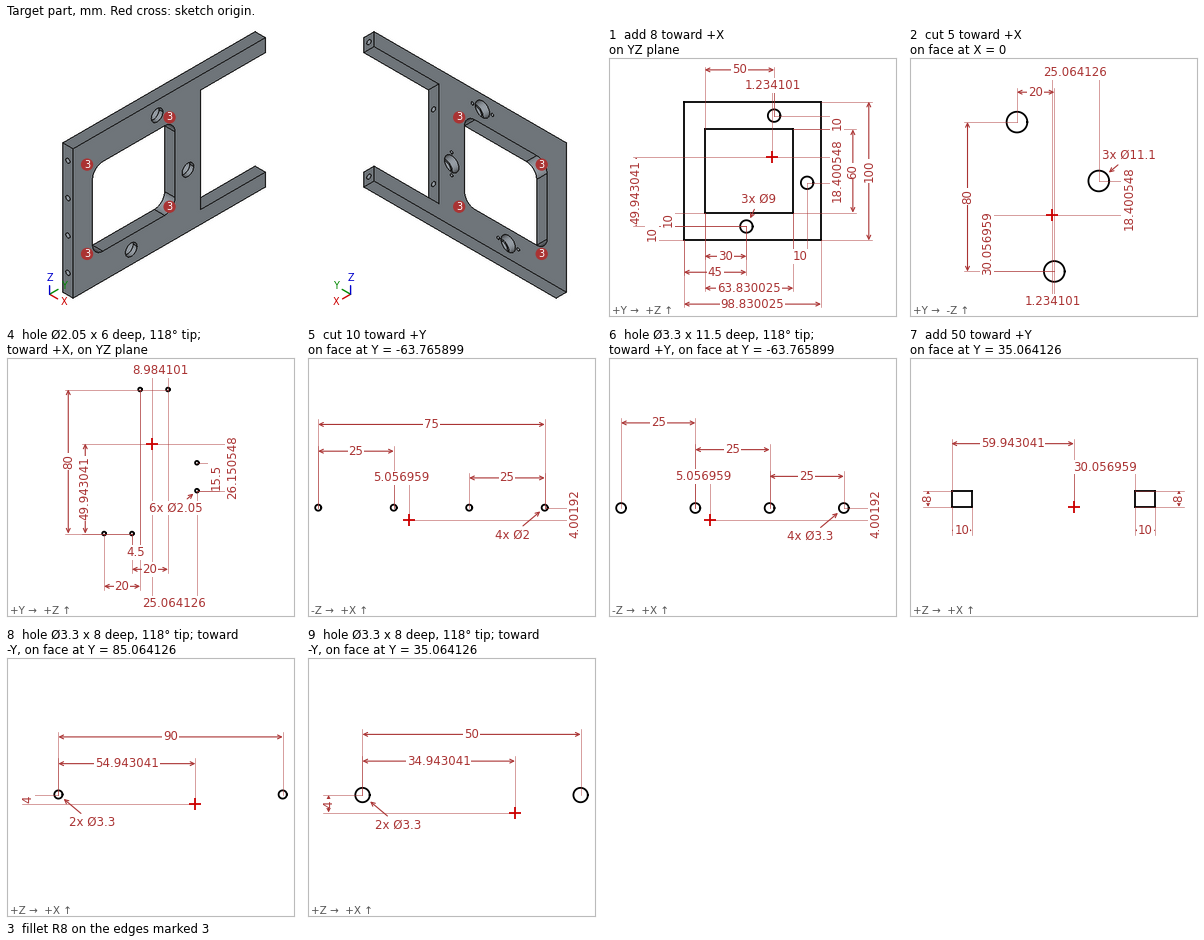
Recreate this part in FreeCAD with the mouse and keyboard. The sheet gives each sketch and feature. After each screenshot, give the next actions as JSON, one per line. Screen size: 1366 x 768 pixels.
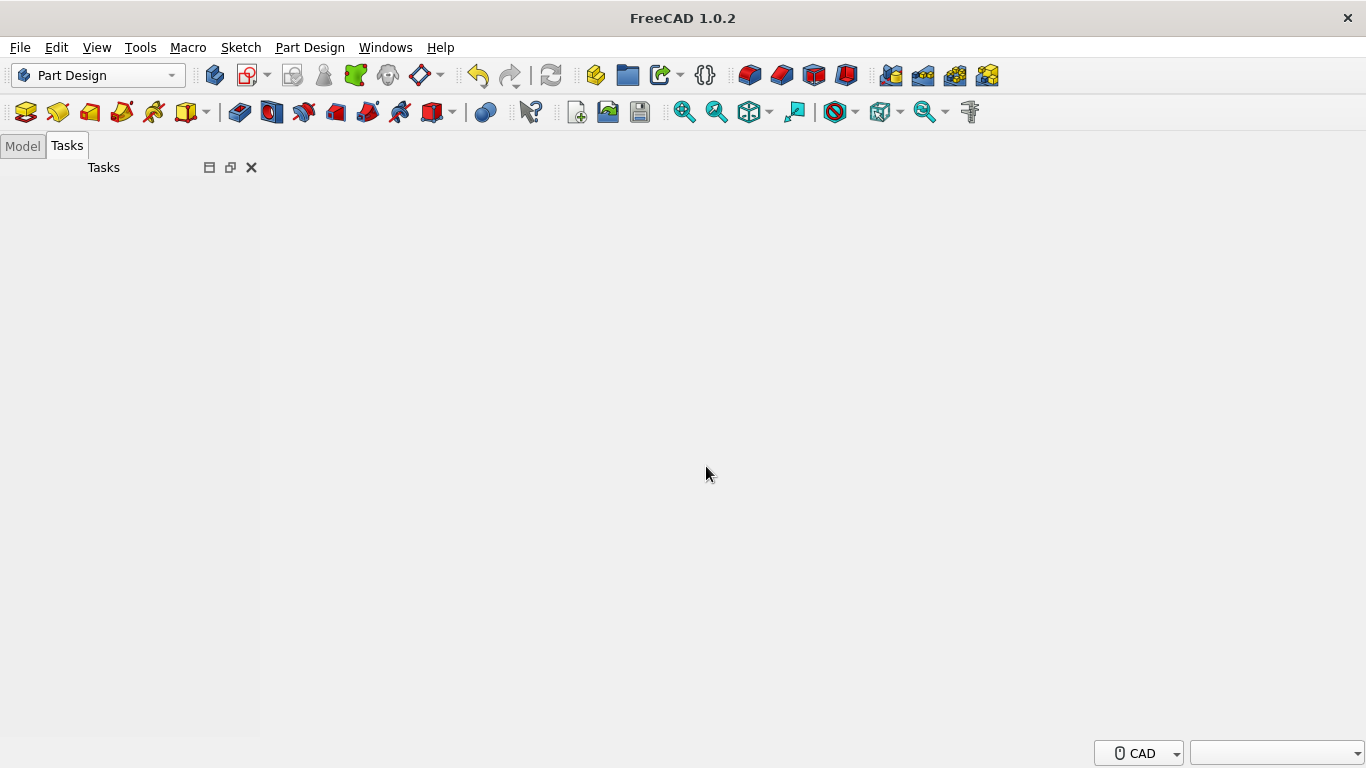
{"action": "left_click", "coordinate": [576, 112]}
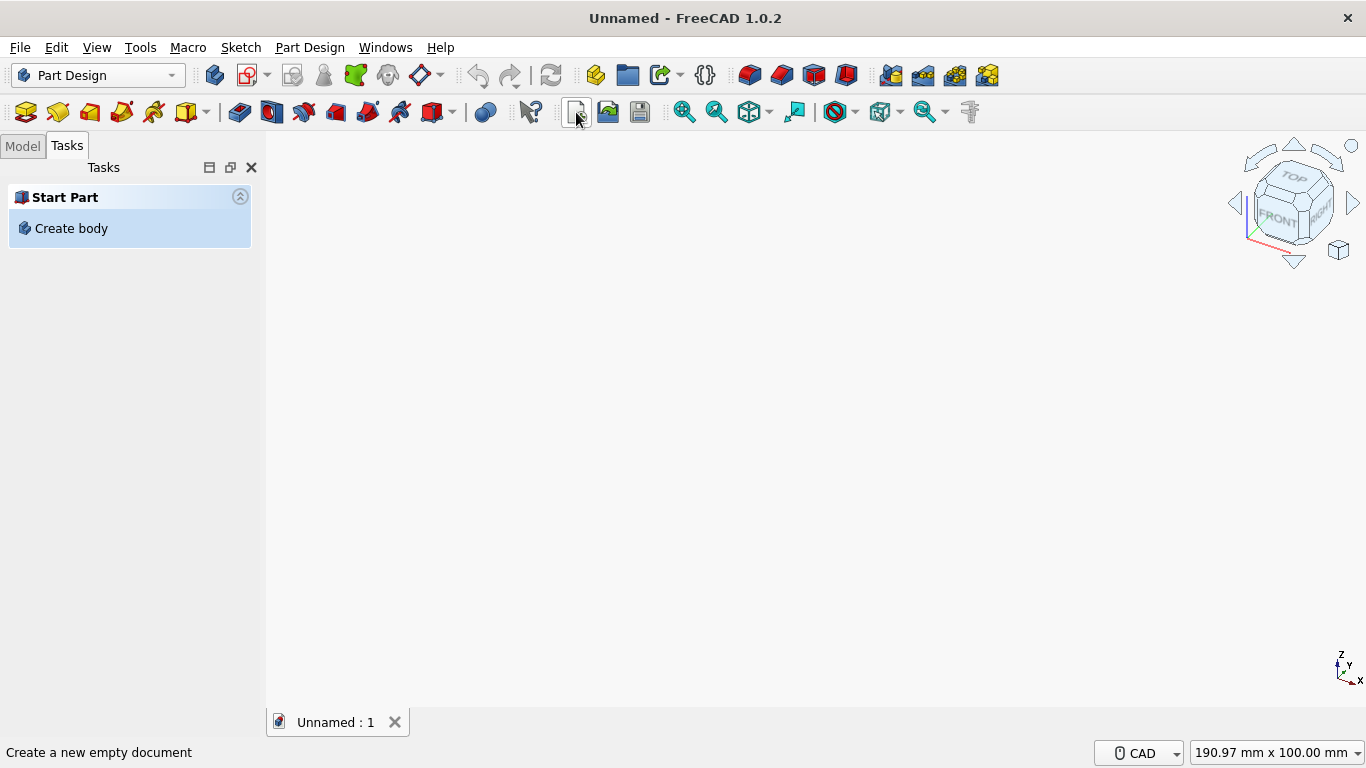
{"action": "left_click", "coordinate": [248, 76]}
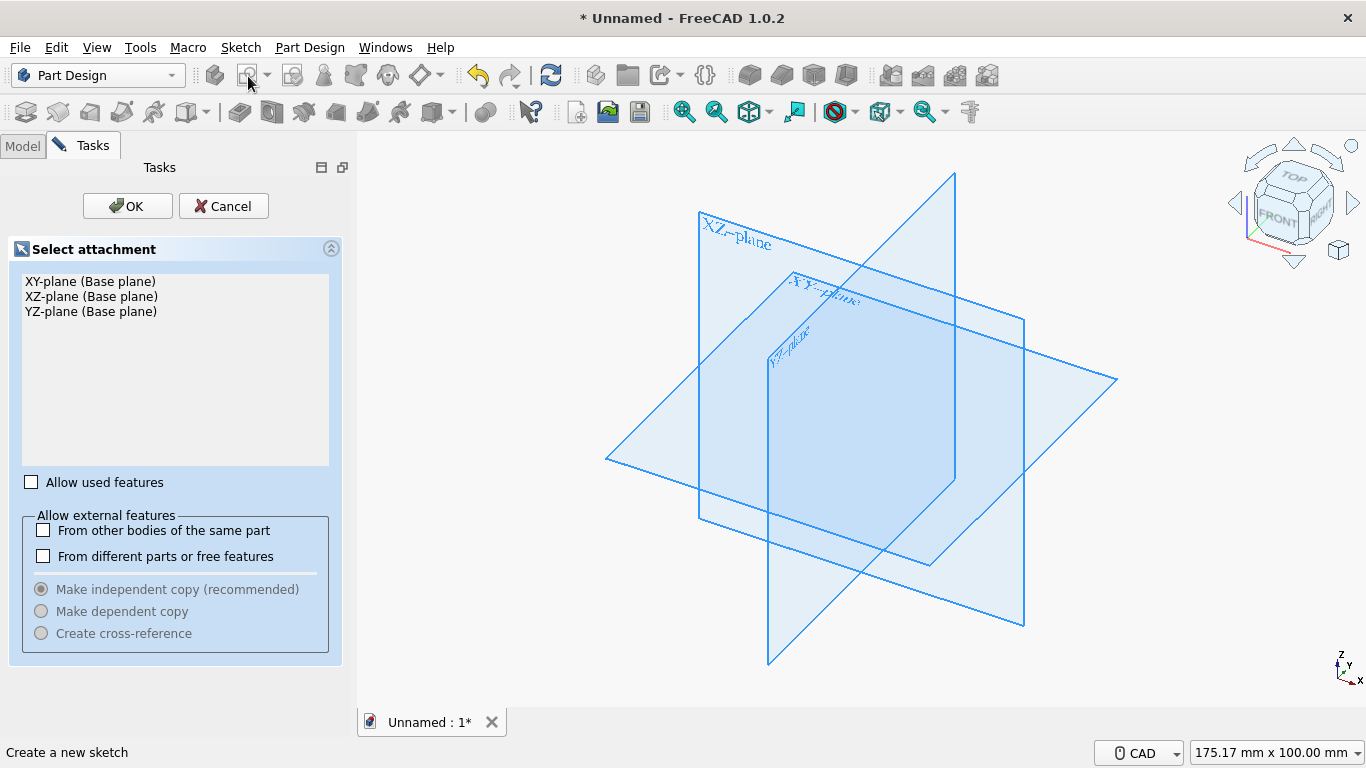
{"action": "left_click", "coordinate": [82, 312]}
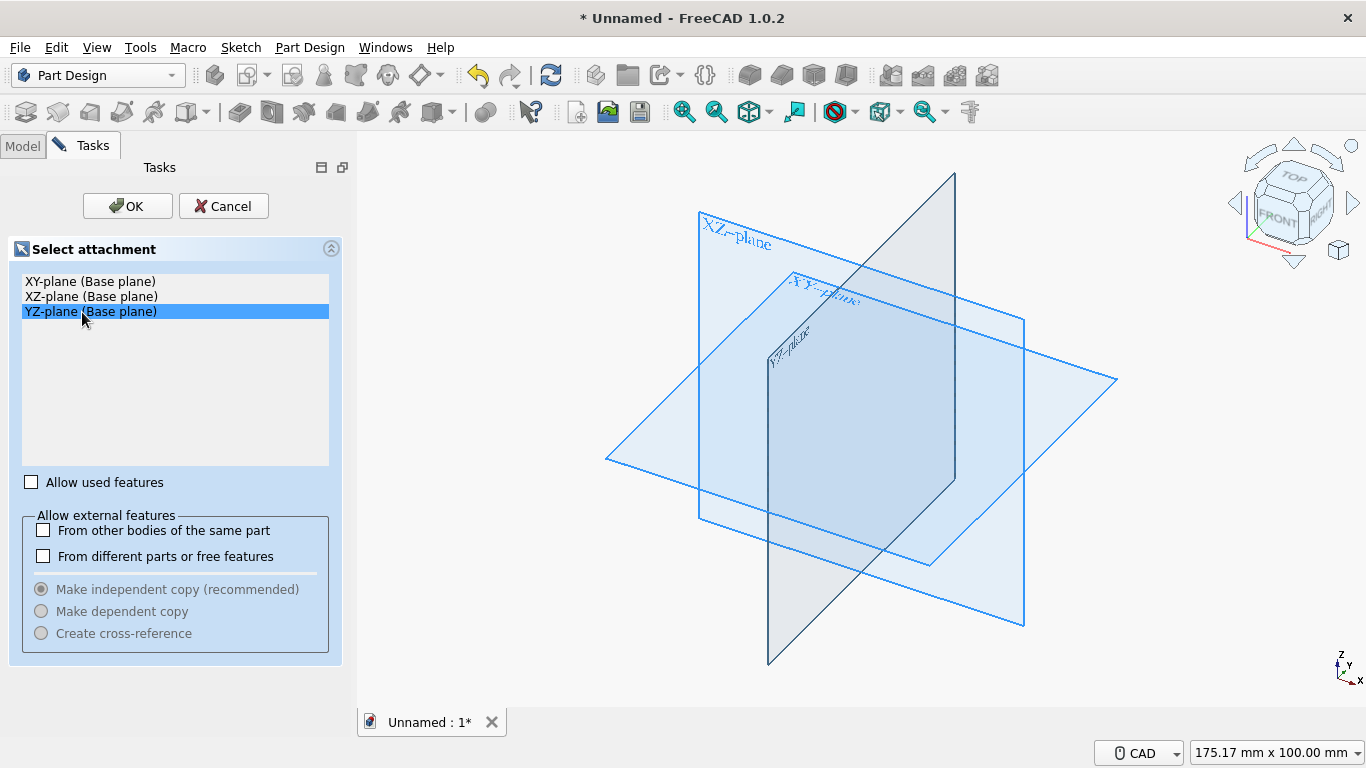
{"action": "left_click", "coordinate": [128, 206]}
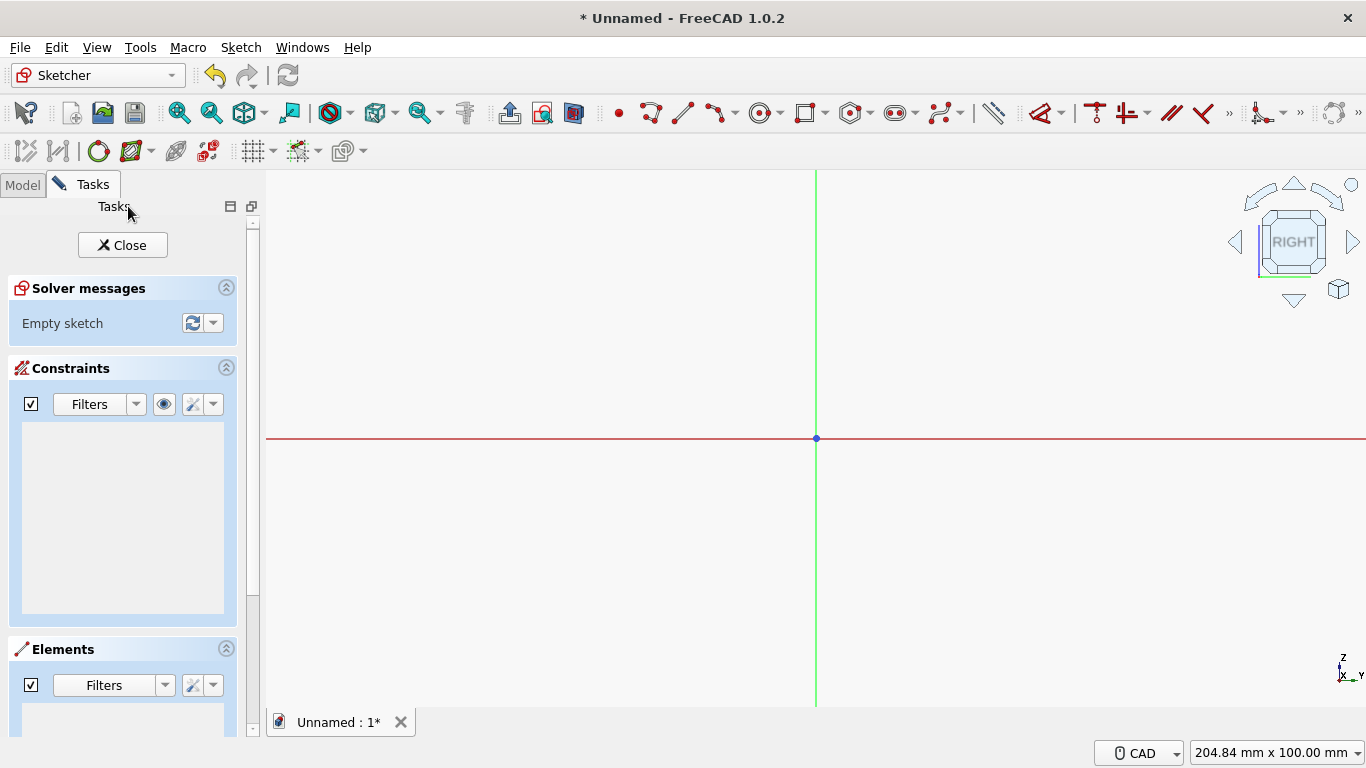
{"action": "scroll", "coordinate": [765, 330], "scroll_direction": "down", "scroll_amount": 2}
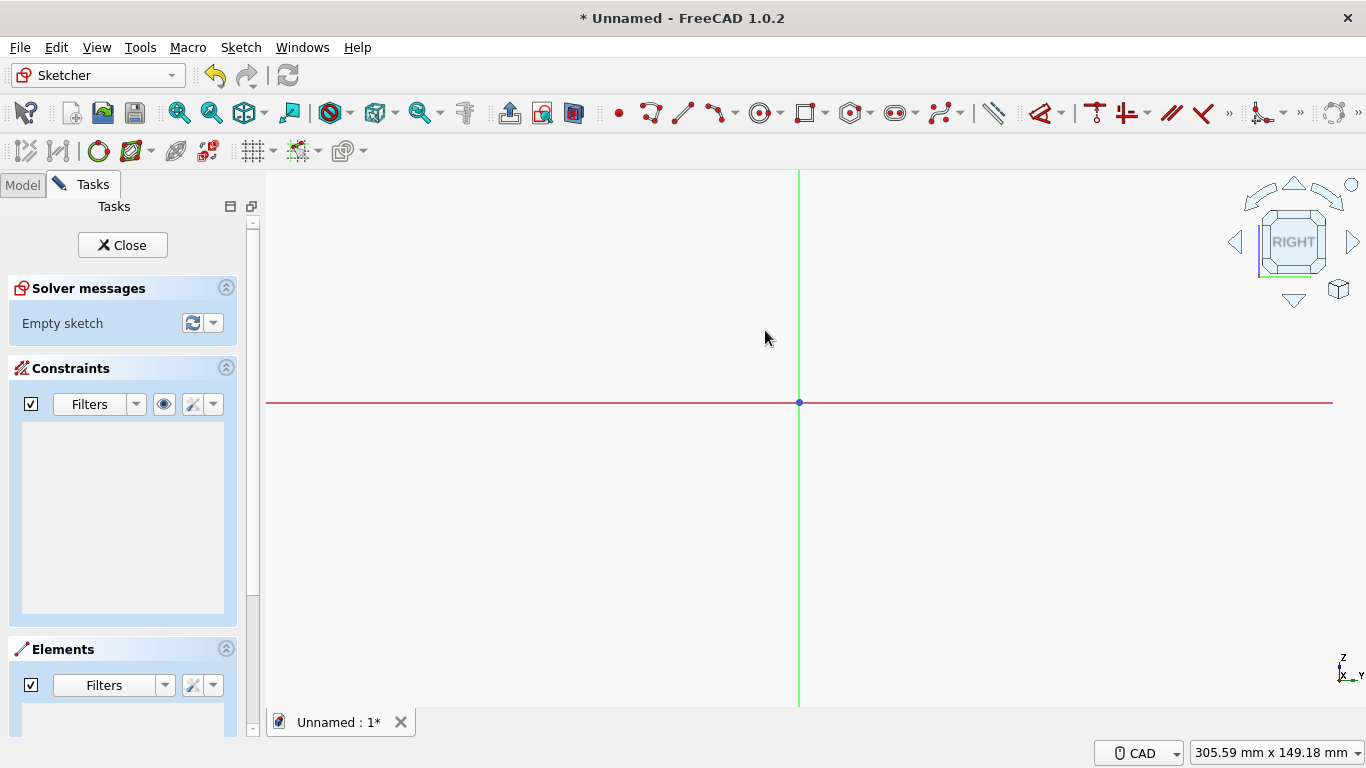
{"action": "left_click", "coordinate": [806, 114]}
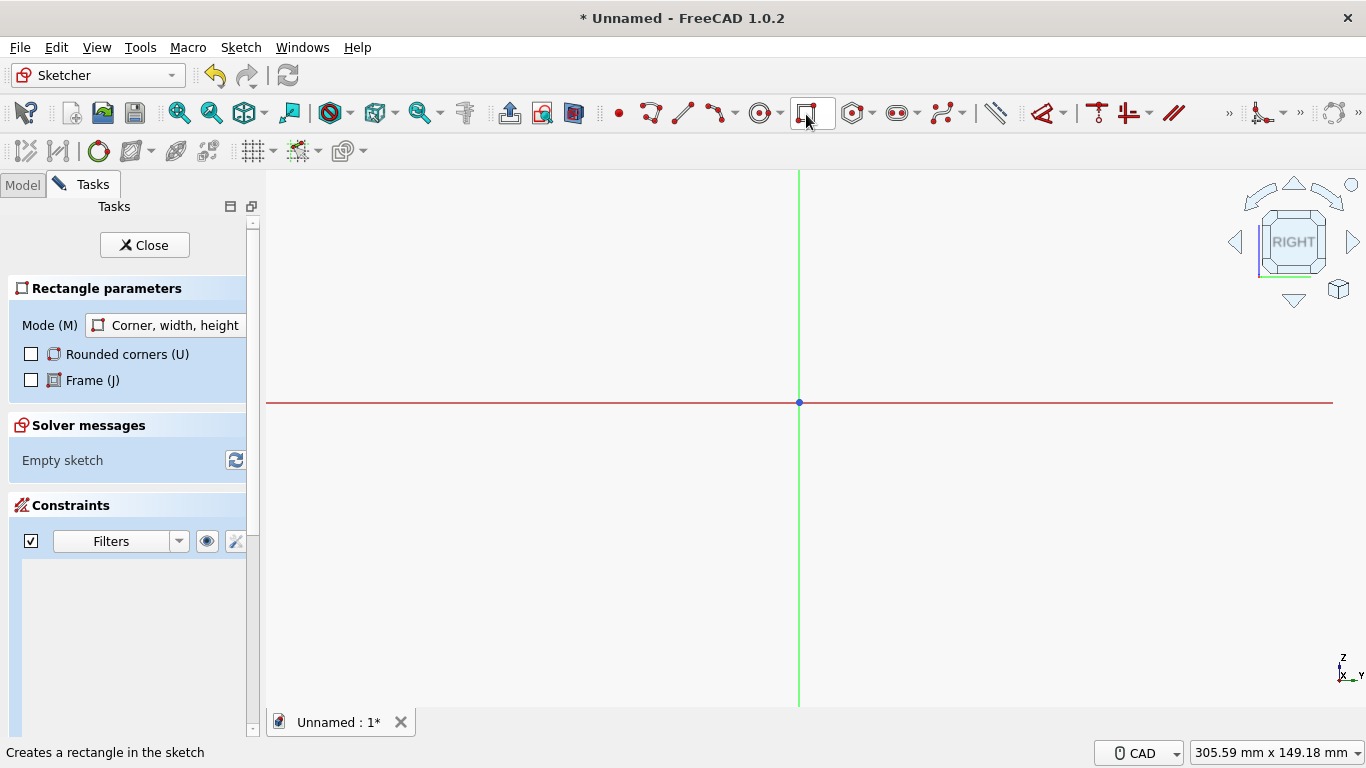
{"action": "left_click", "coordinate": [570, 259]}
{"action": "mouse_move", "coordinate": [926, 619]}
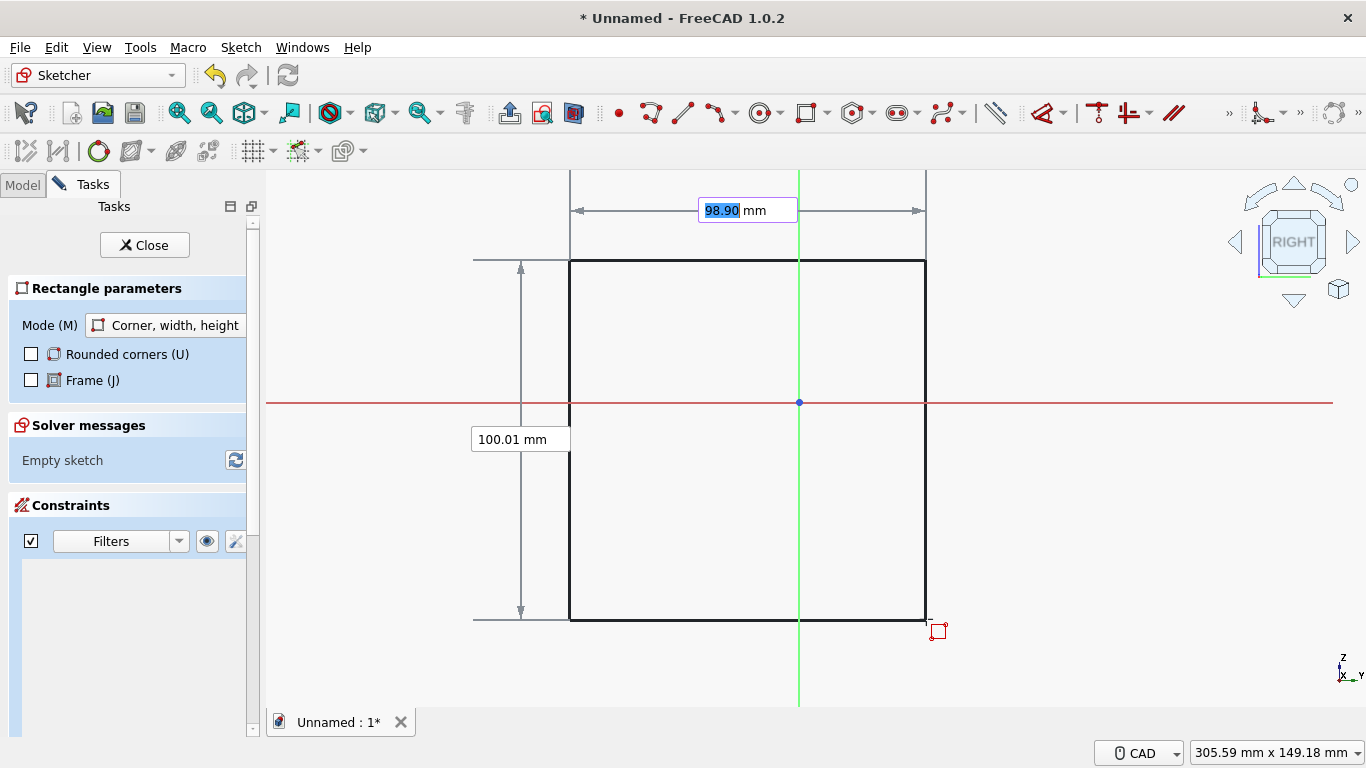
{"action": "type", "text": "98.830025"}
{"action": "key", "text": "Tab"}
{"action": "type", "text": "100"}
{"action": "key", "text": "Return"}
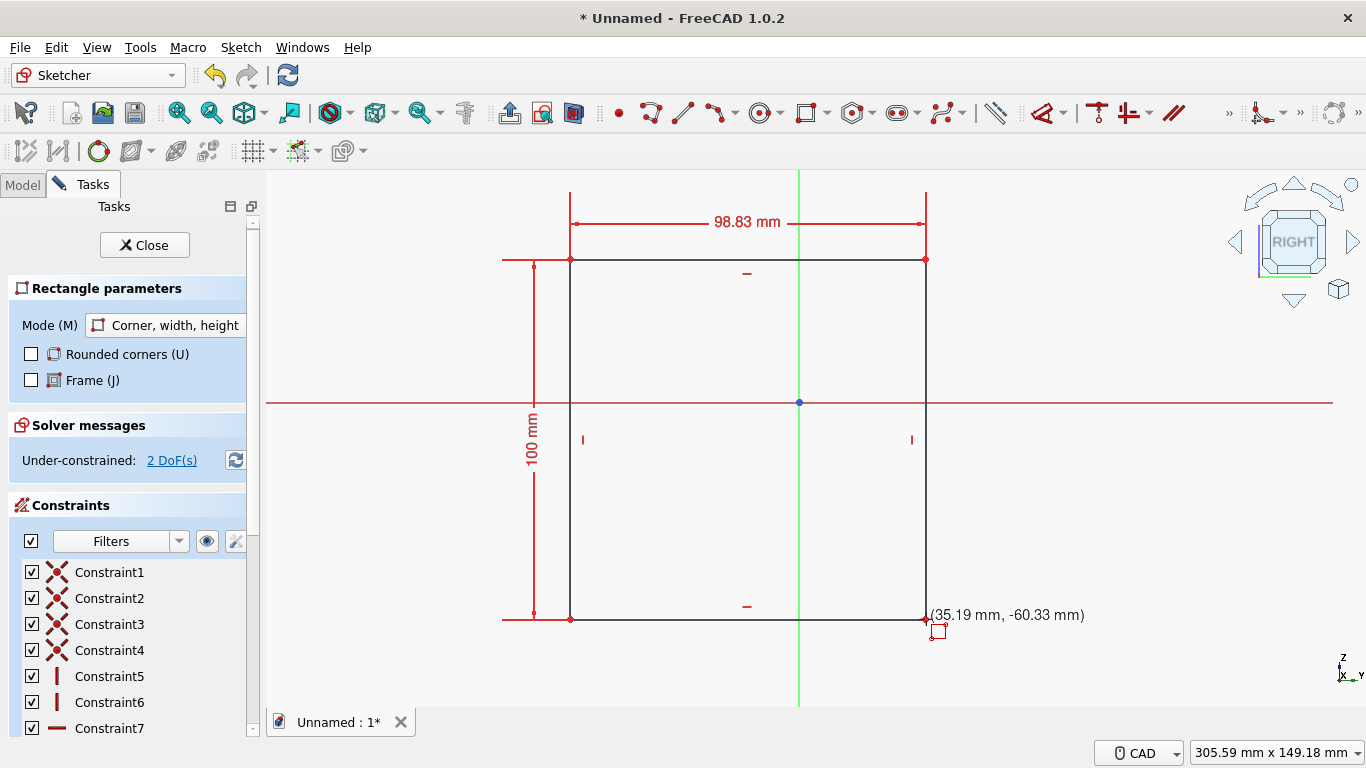
{"action": "left_click", "coordinate": [624, 331]}
{"action": "mouse_move", "coordinate": [854, 547]}